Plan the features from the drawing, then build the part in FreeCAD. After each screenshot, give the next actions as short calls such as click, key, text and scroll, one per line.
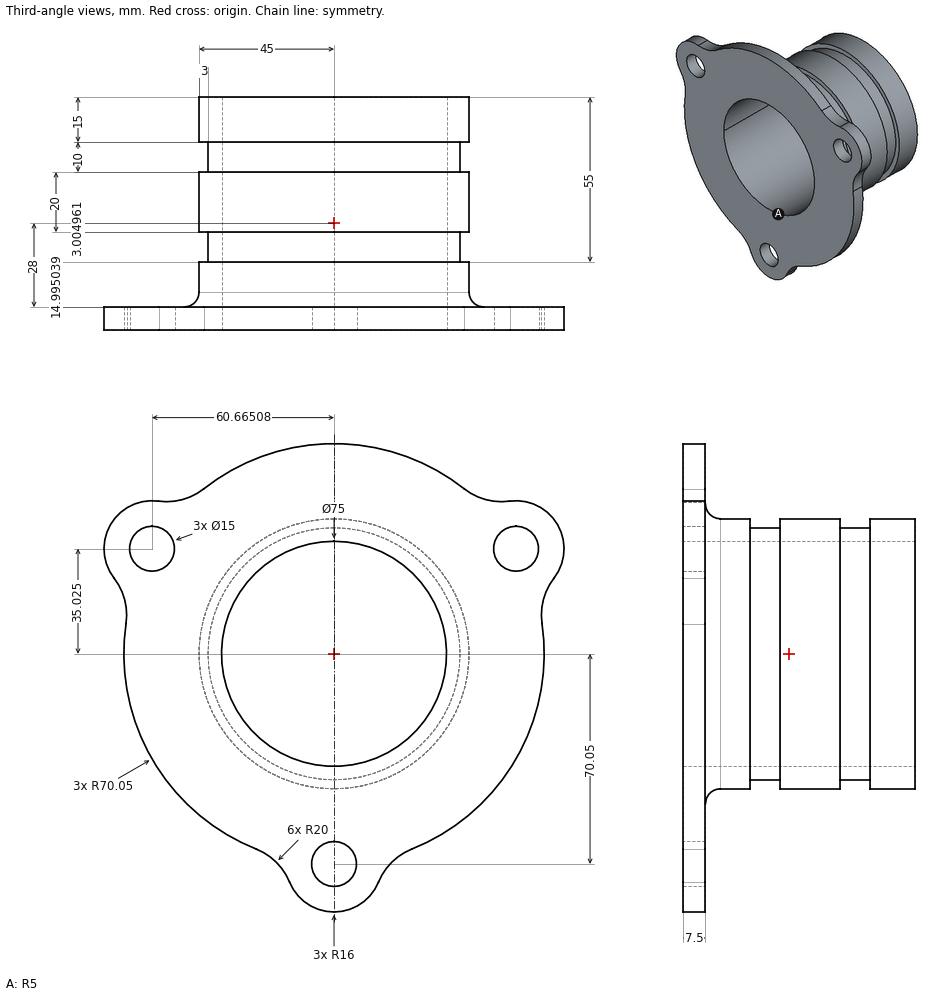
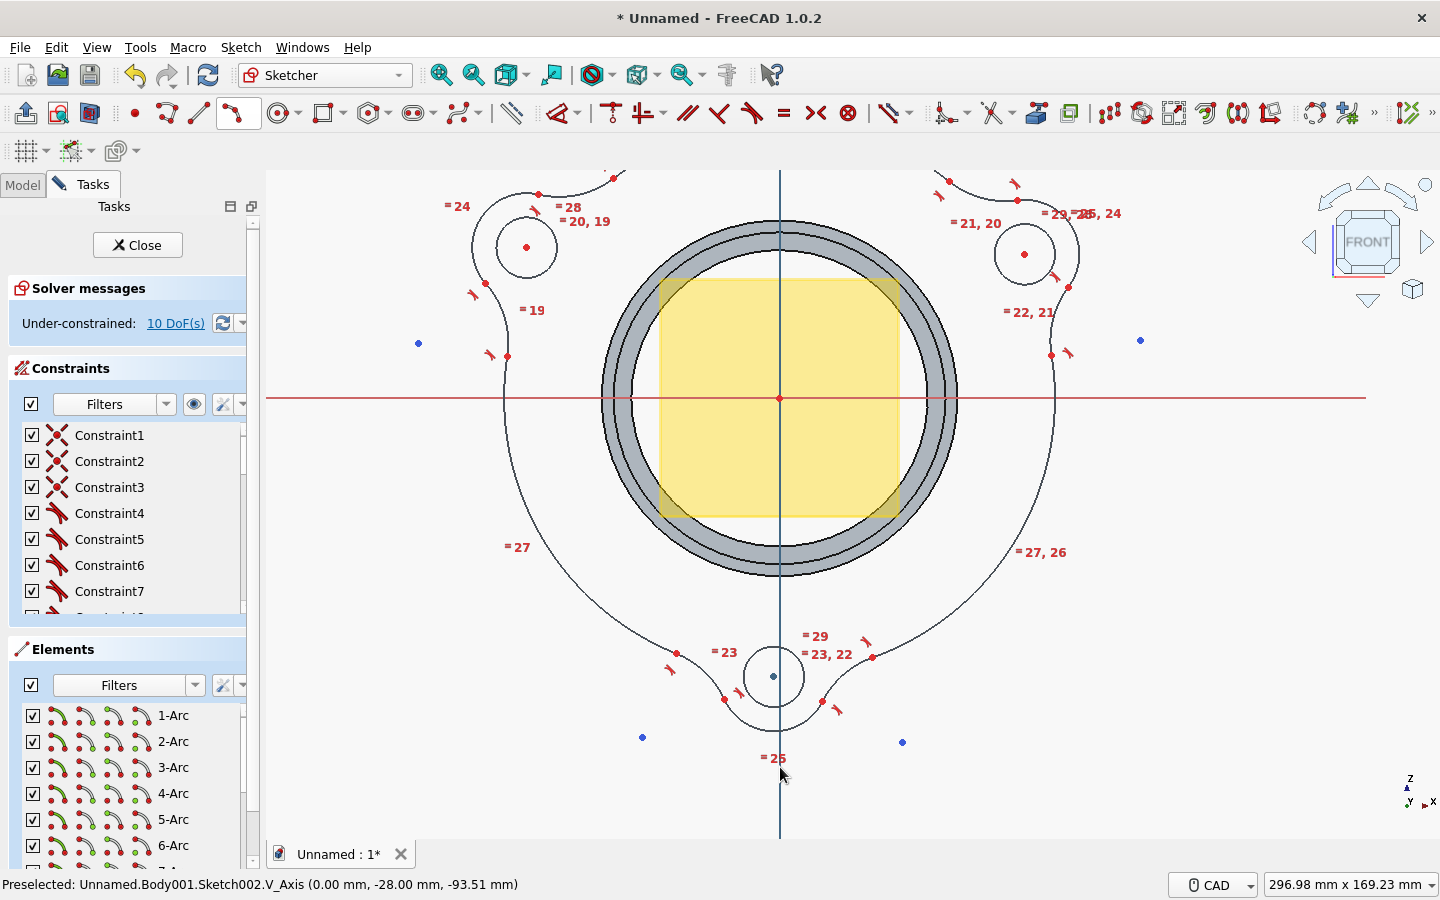
key(c)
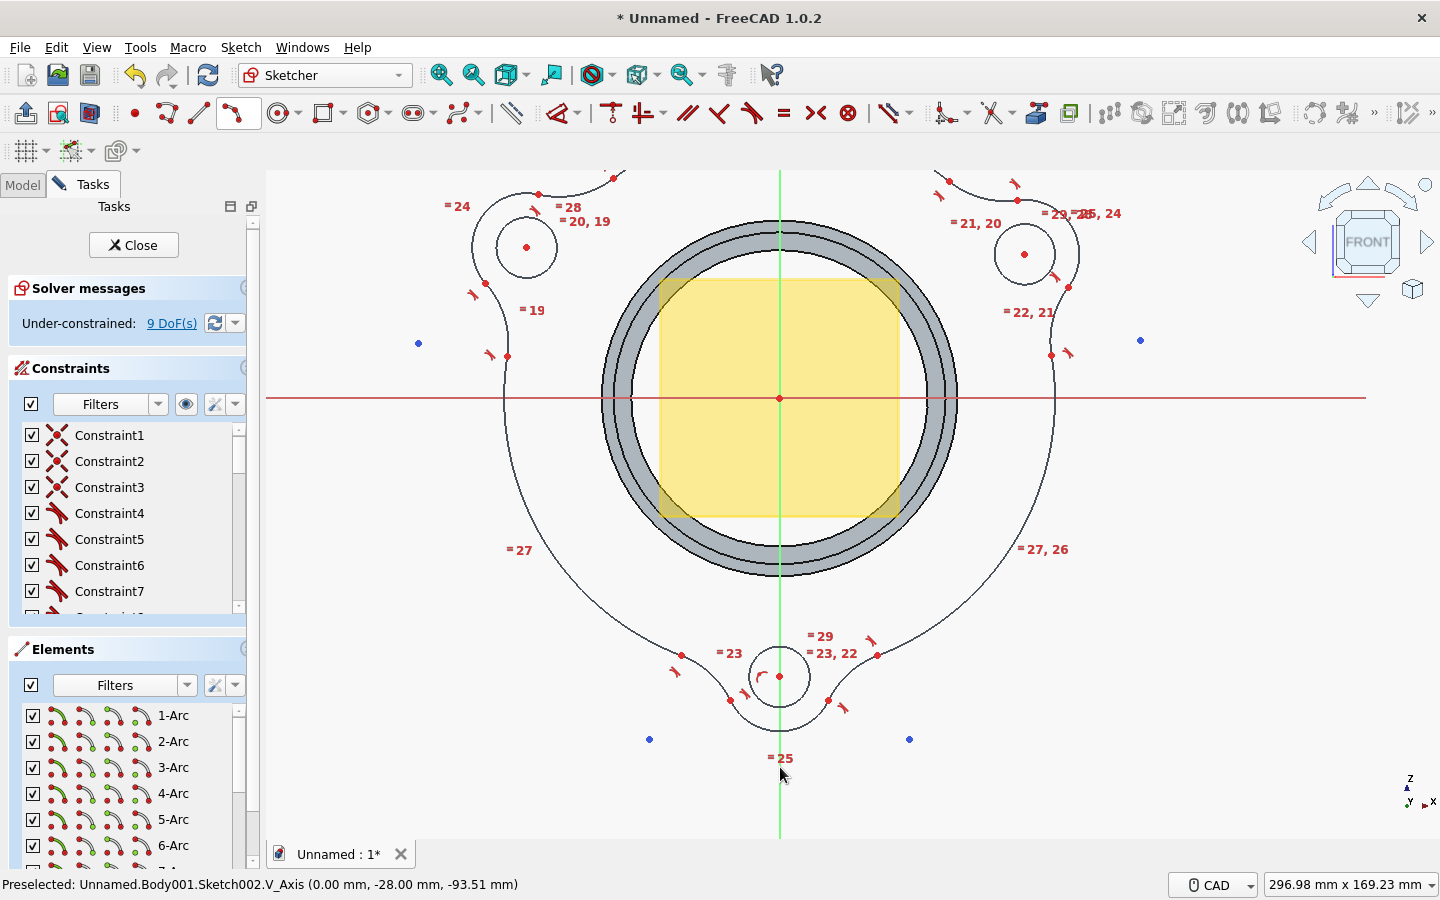
click(527, 248)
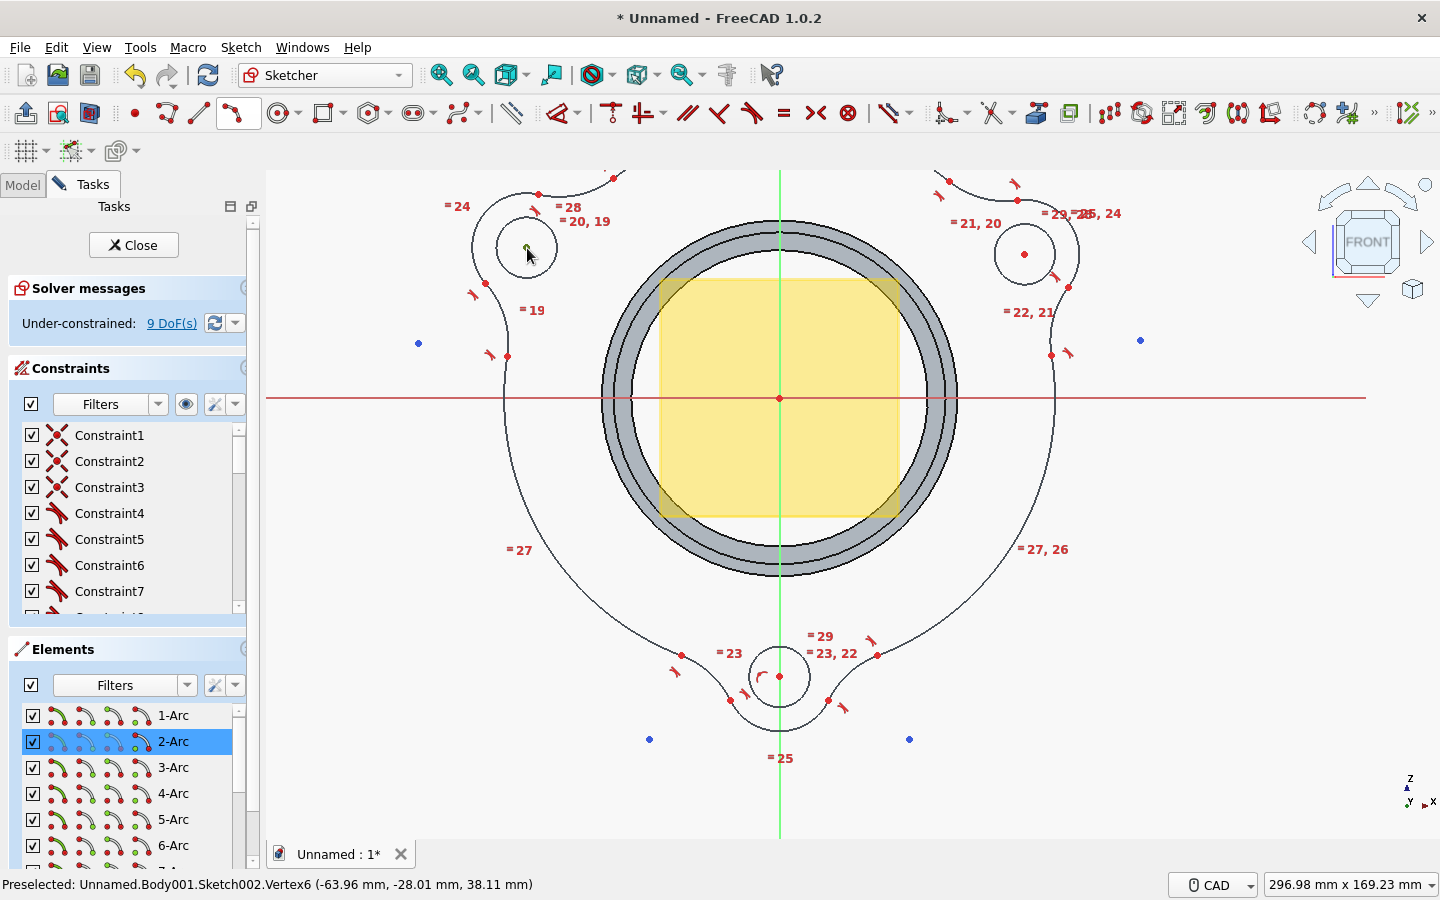
click(1025, 254)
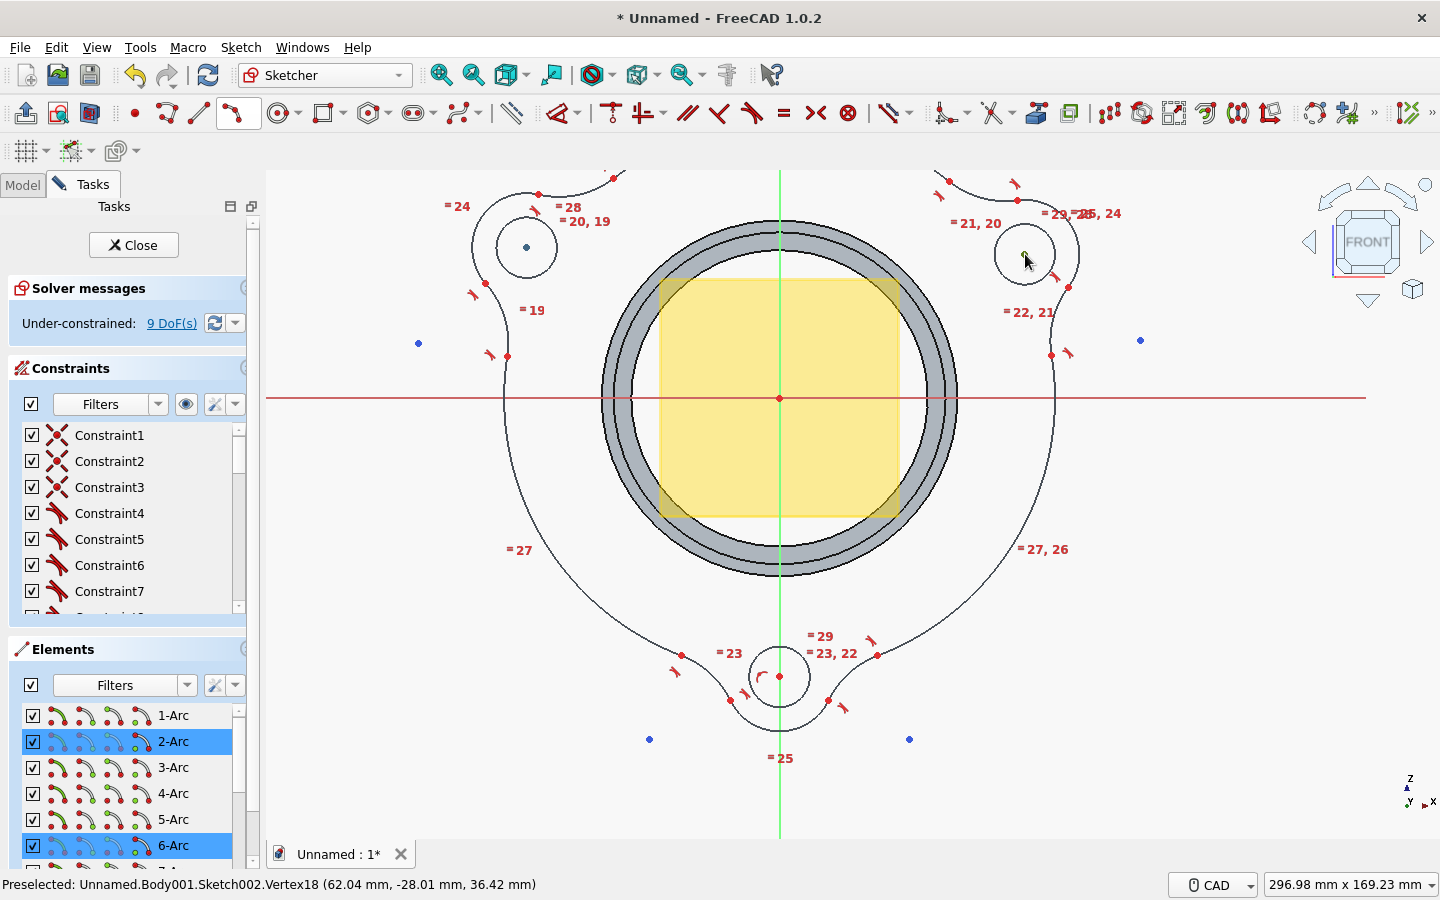
click(780, 767)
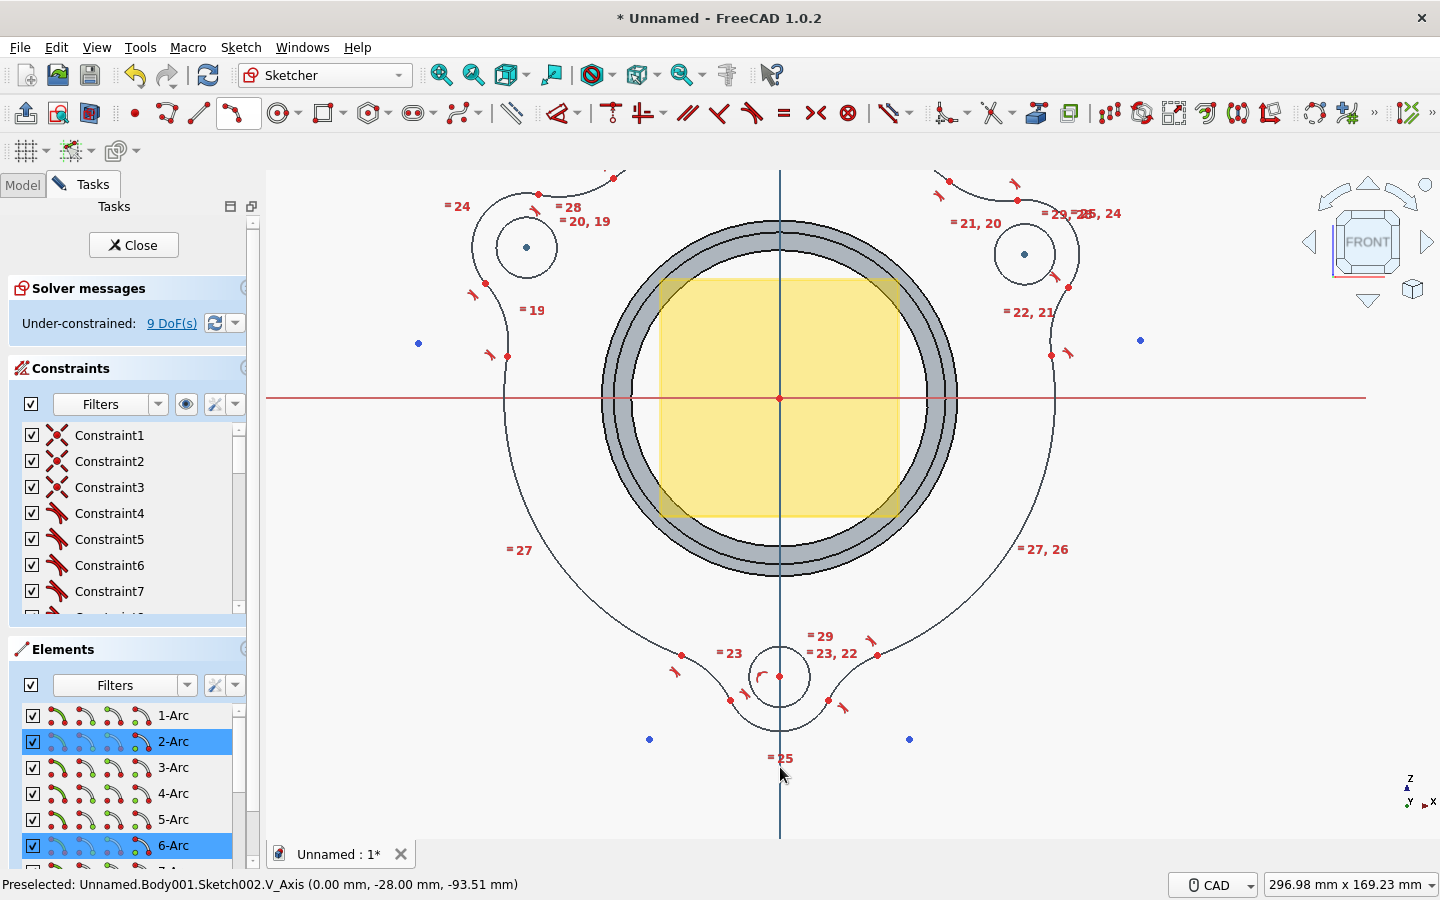
key(s)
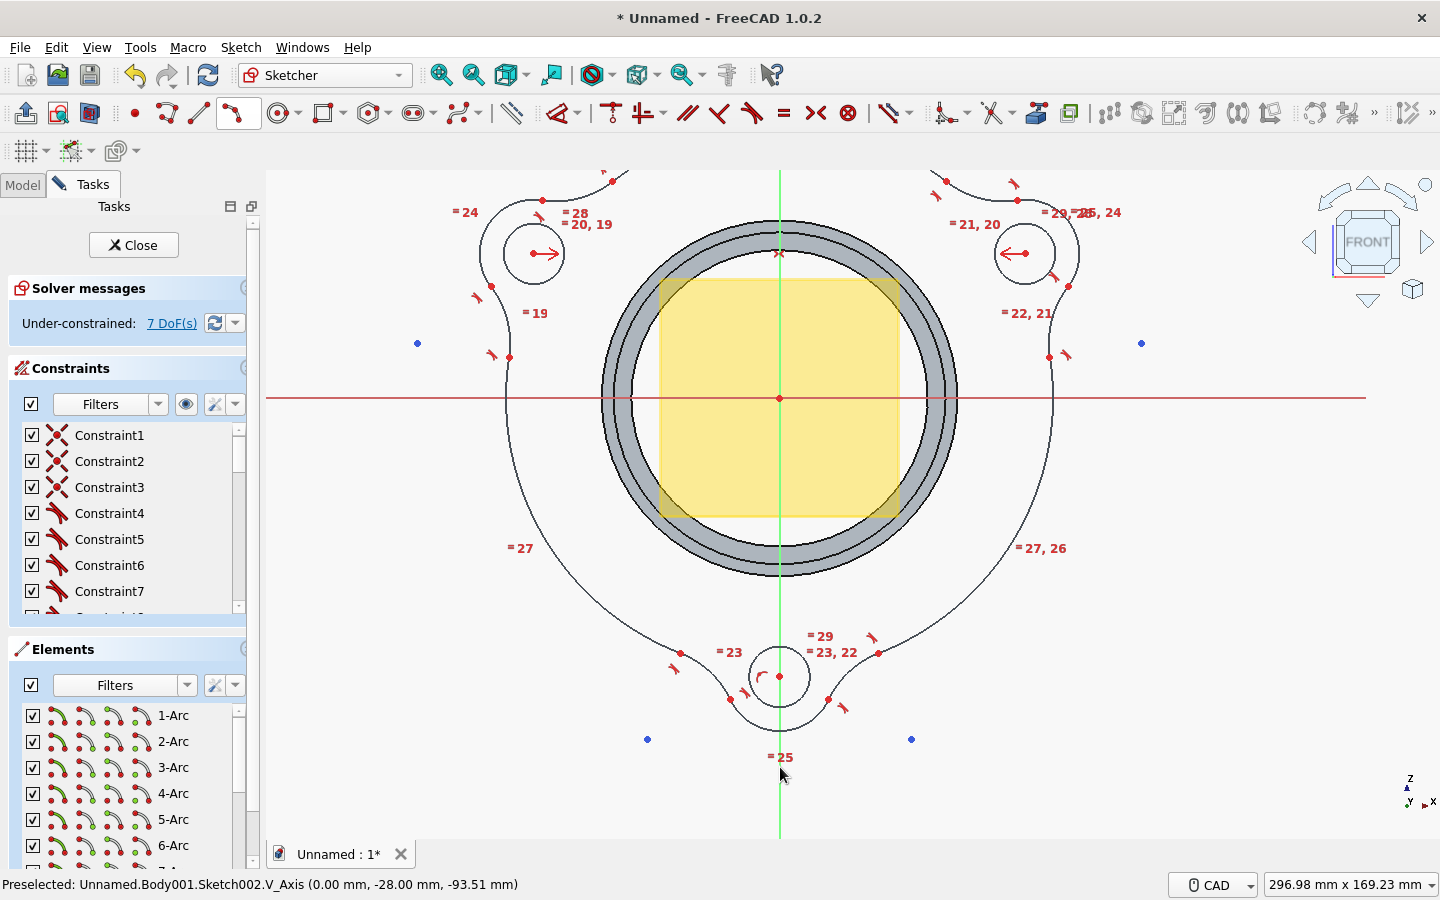
key(d)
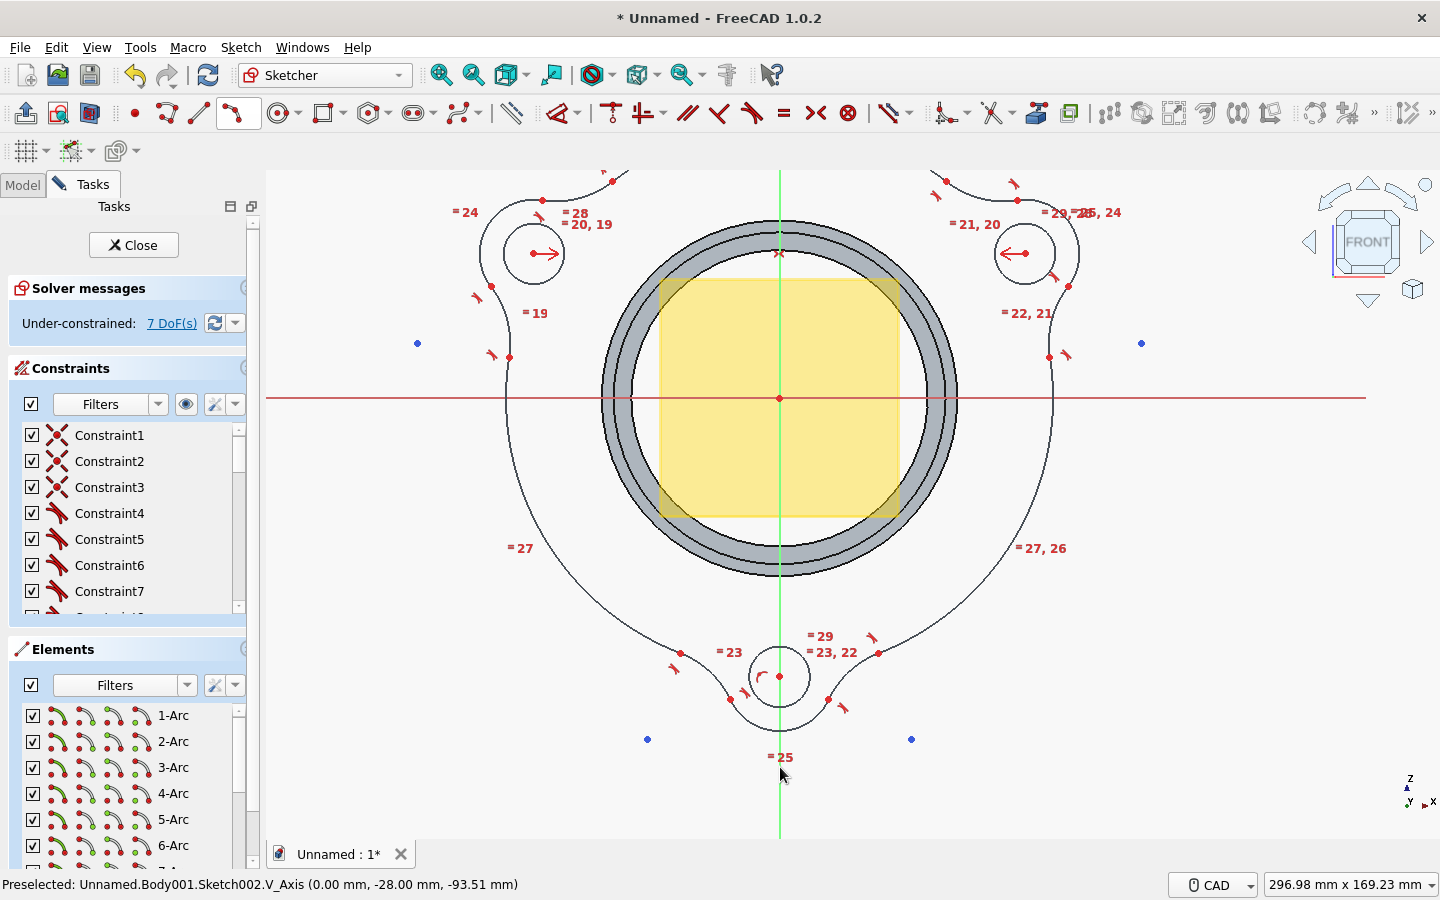
click(510, 335)
click(542, 332)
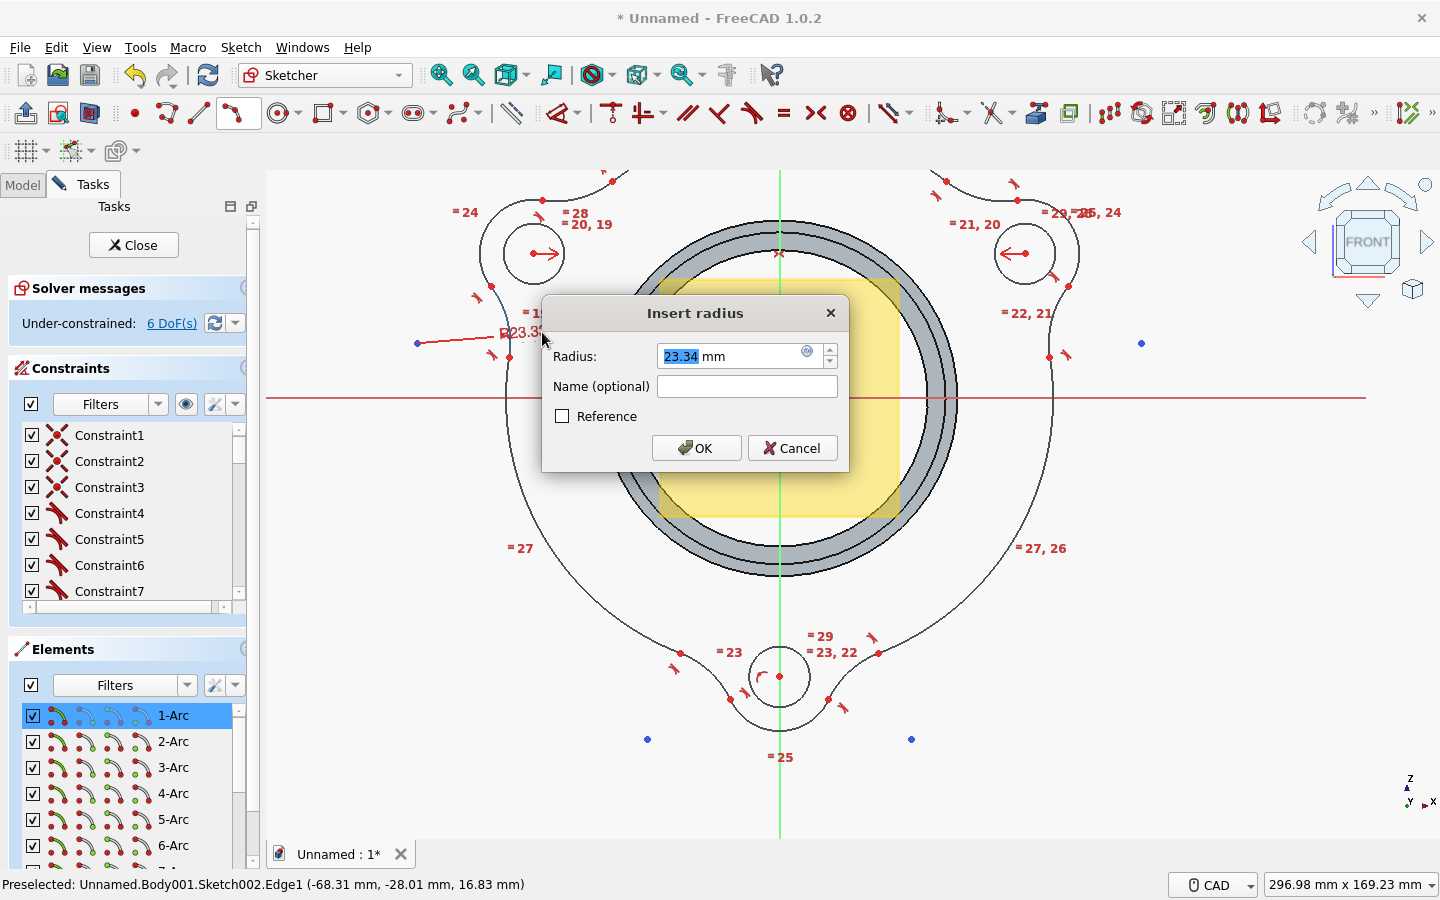
text(20)
key(Return)